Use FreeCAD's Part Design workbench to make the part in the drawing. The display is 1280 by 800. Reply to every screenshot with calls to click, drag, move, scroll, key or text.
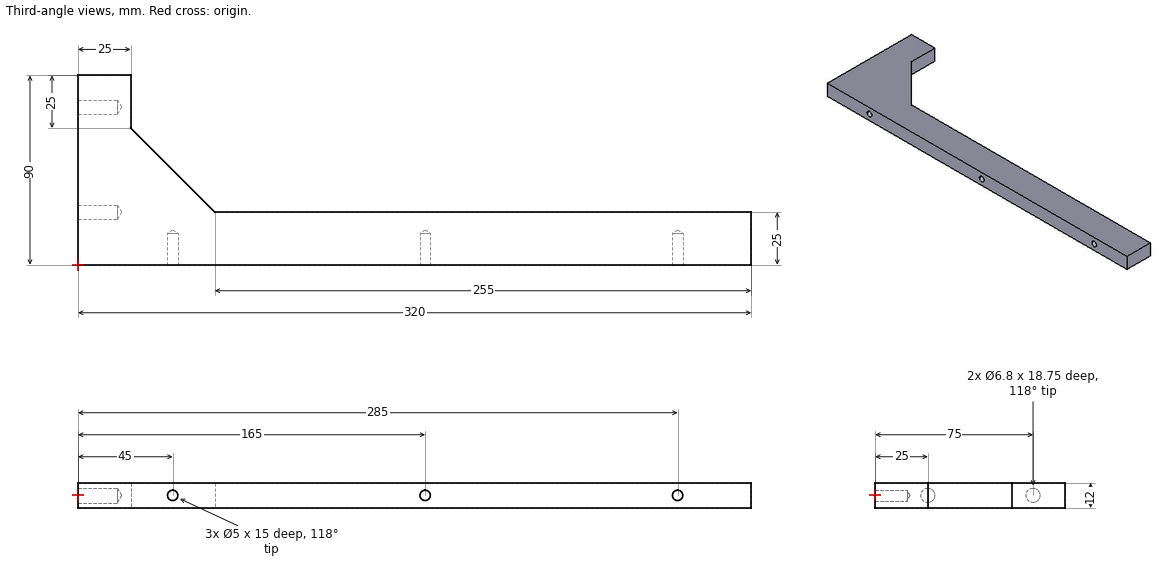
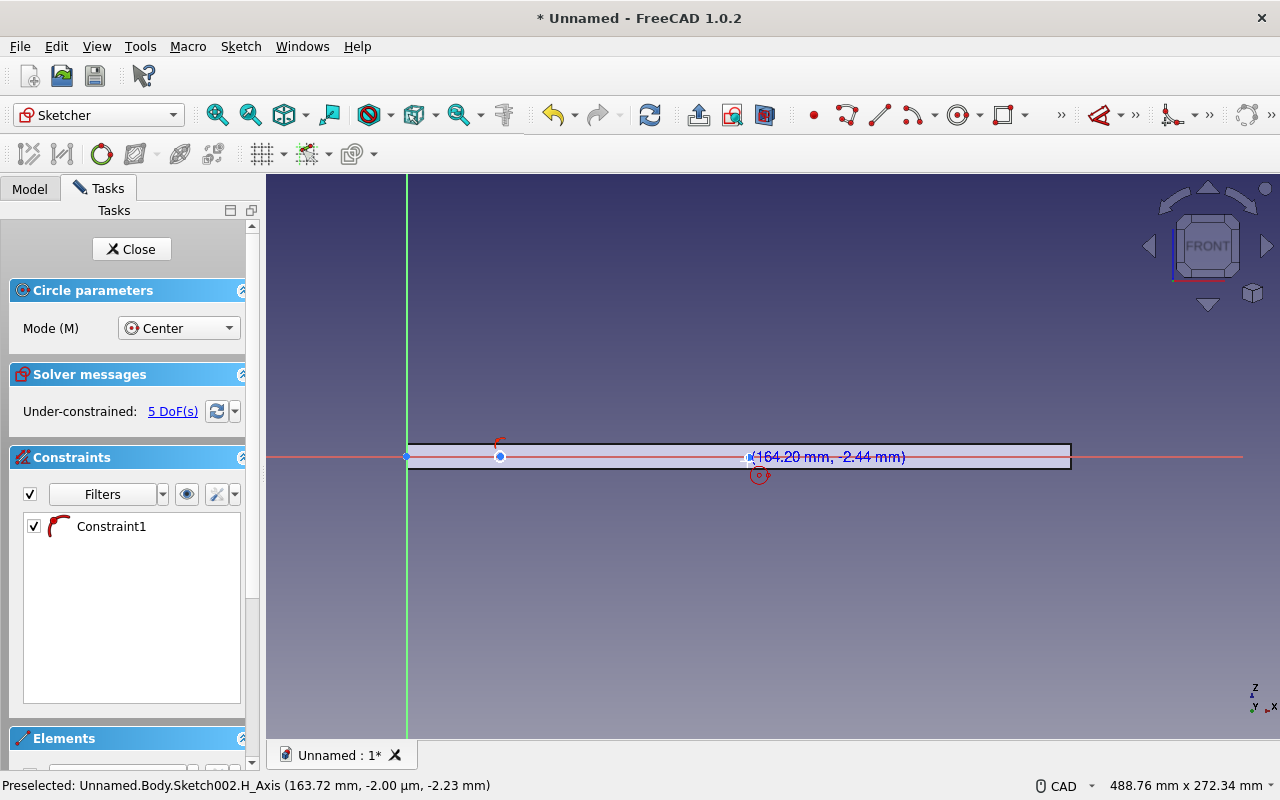
scroll(998, 457, up, 8)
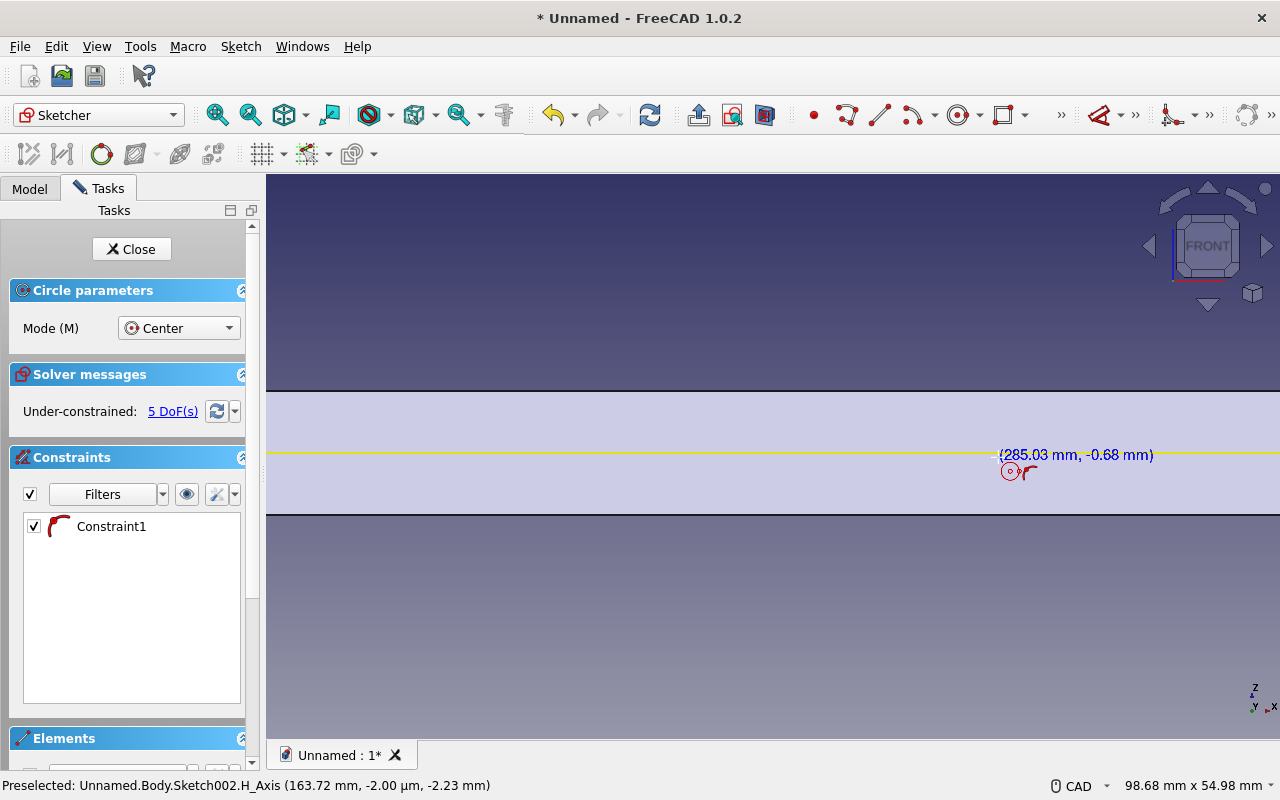
scroll(998, 457, down, 8)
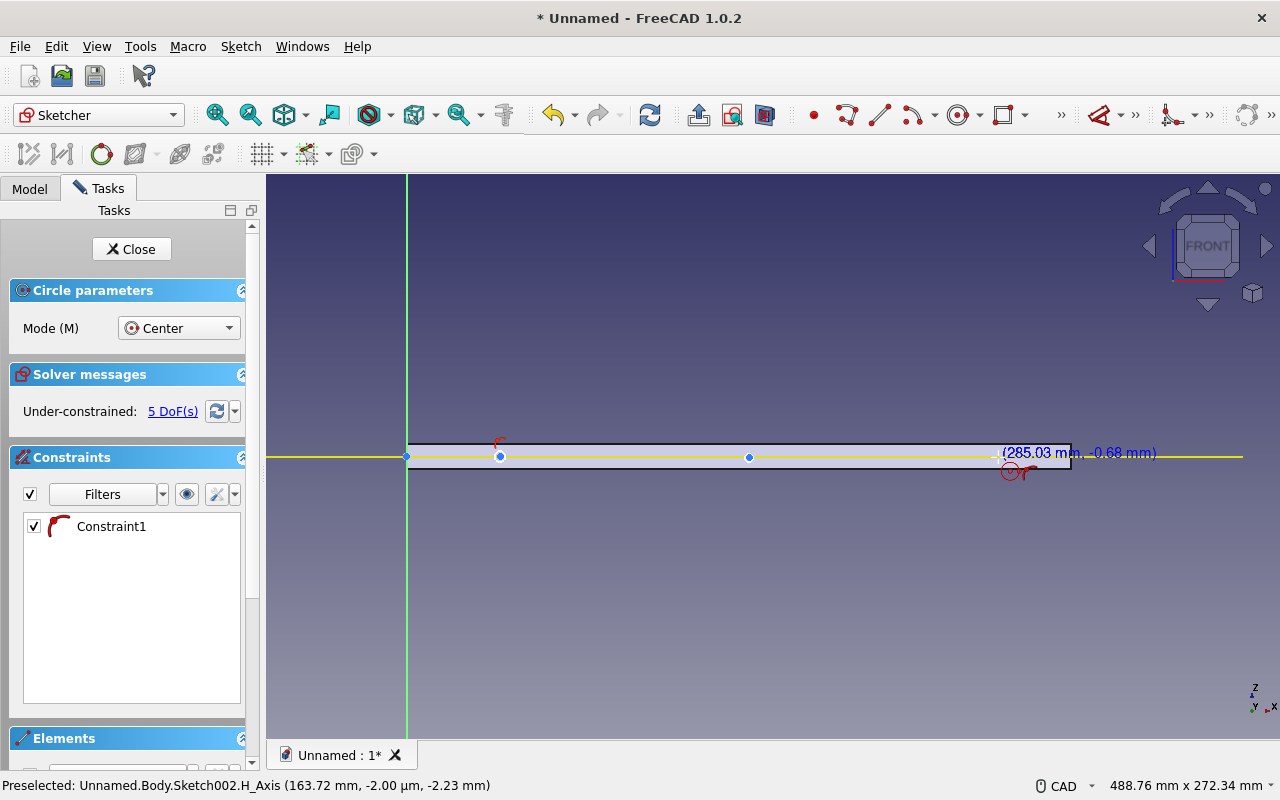
click(998, 457)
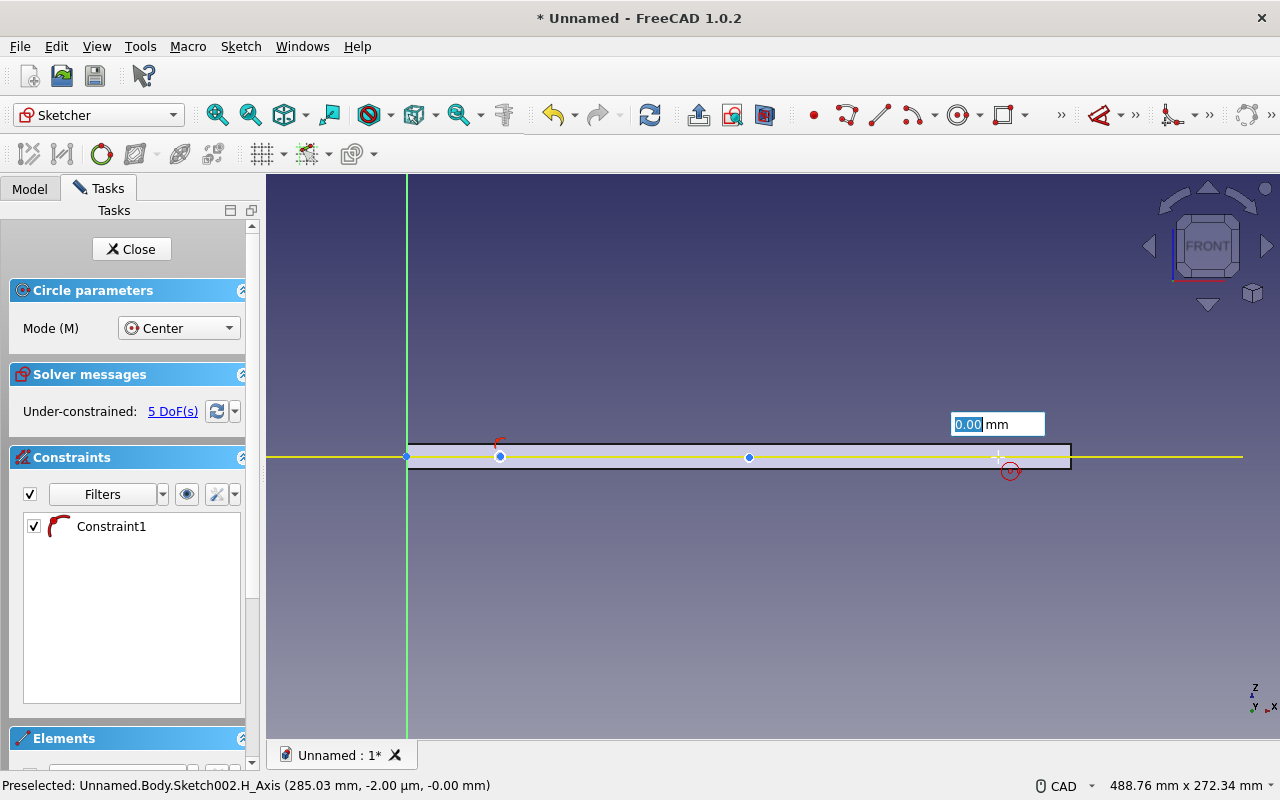
scroll(996, 461, up, 6)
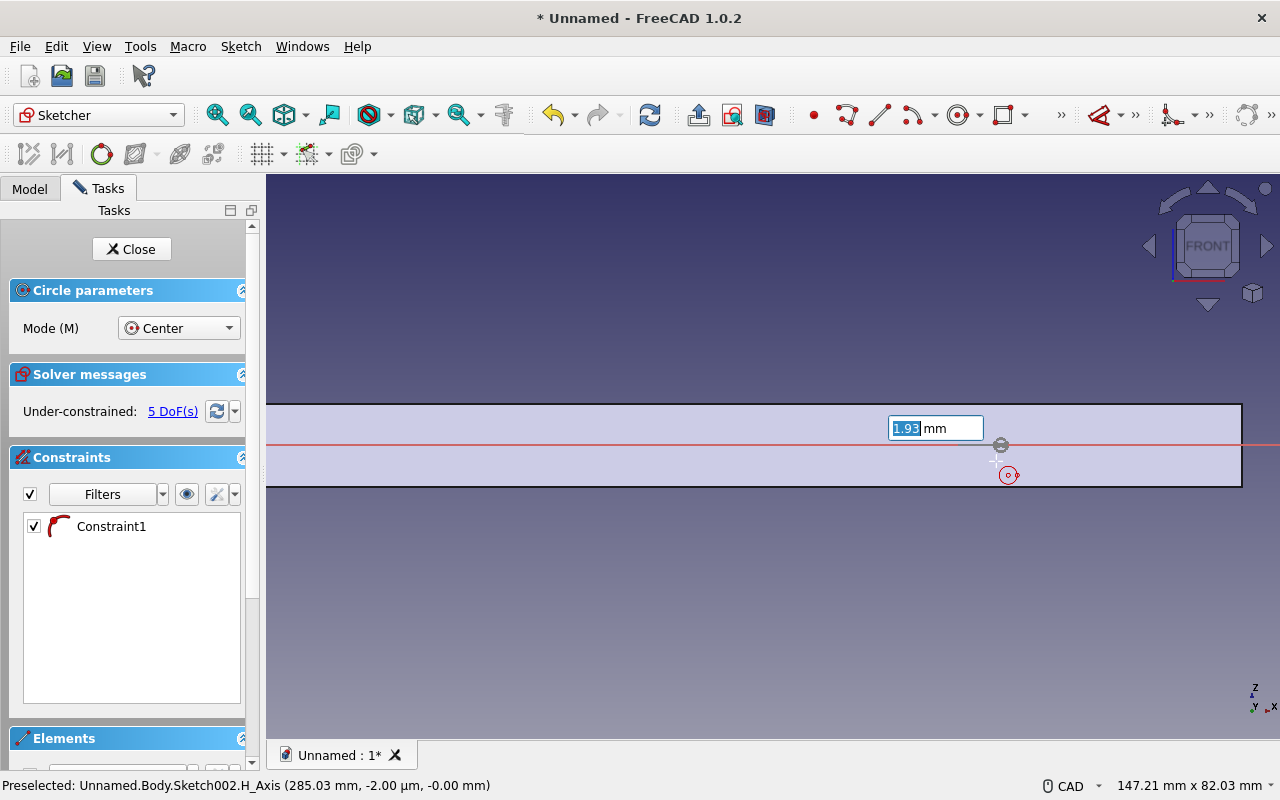
click(995, 461)
key(Escape)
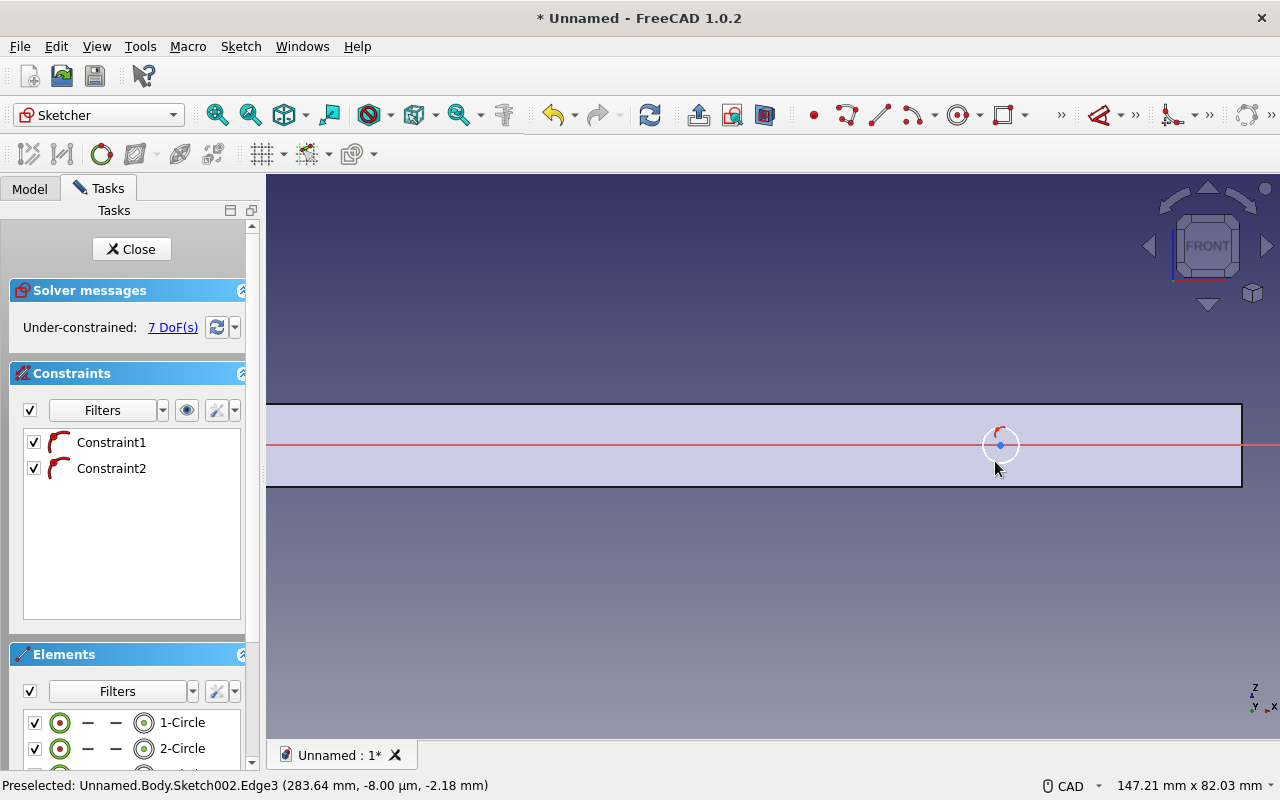
scroll(996, 461, down, 6)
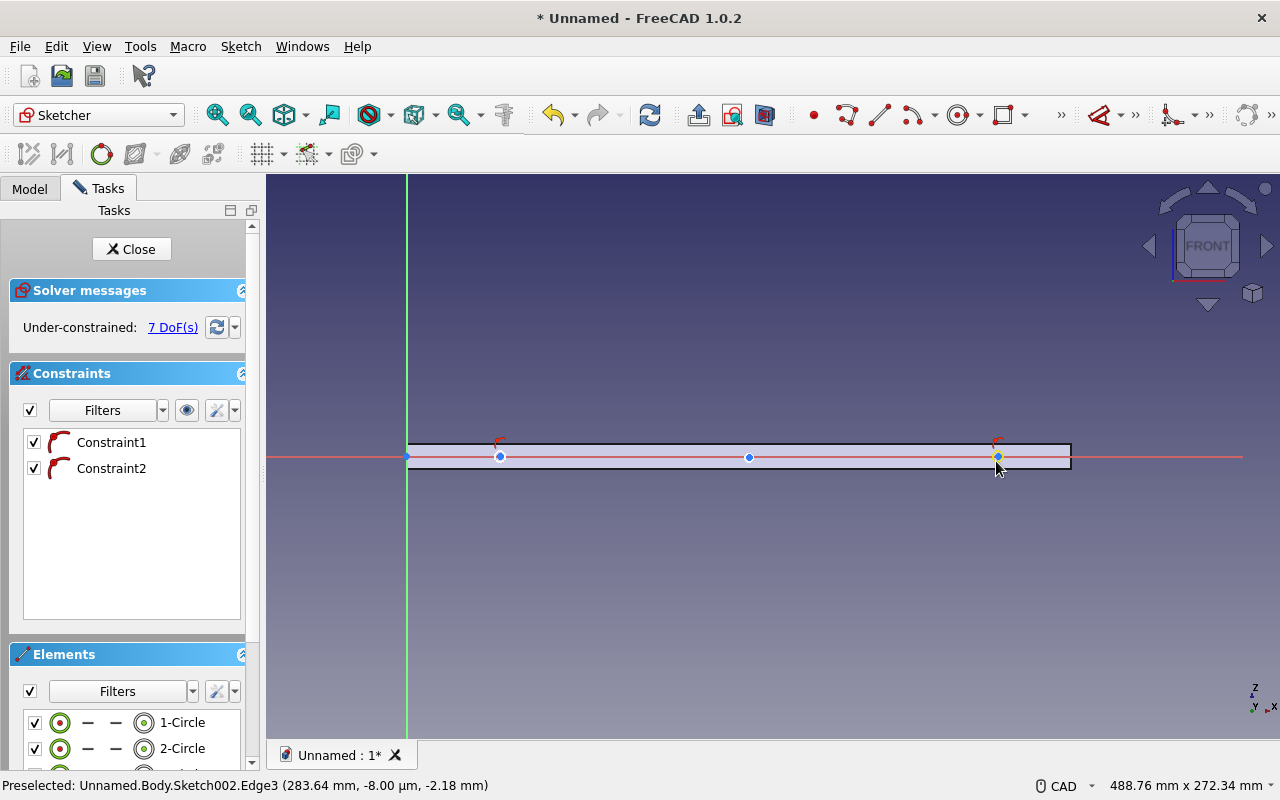
scroll(504, 453, up, 7)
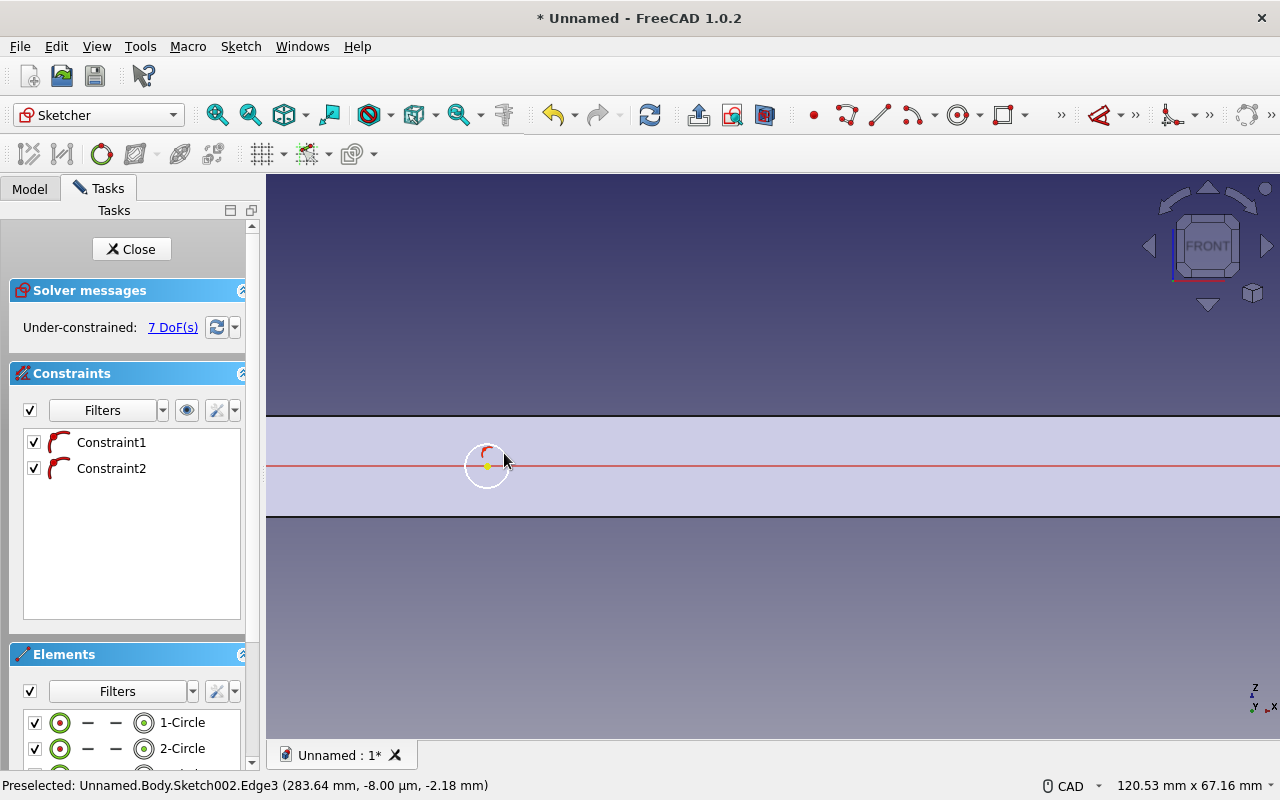
click(502, 451)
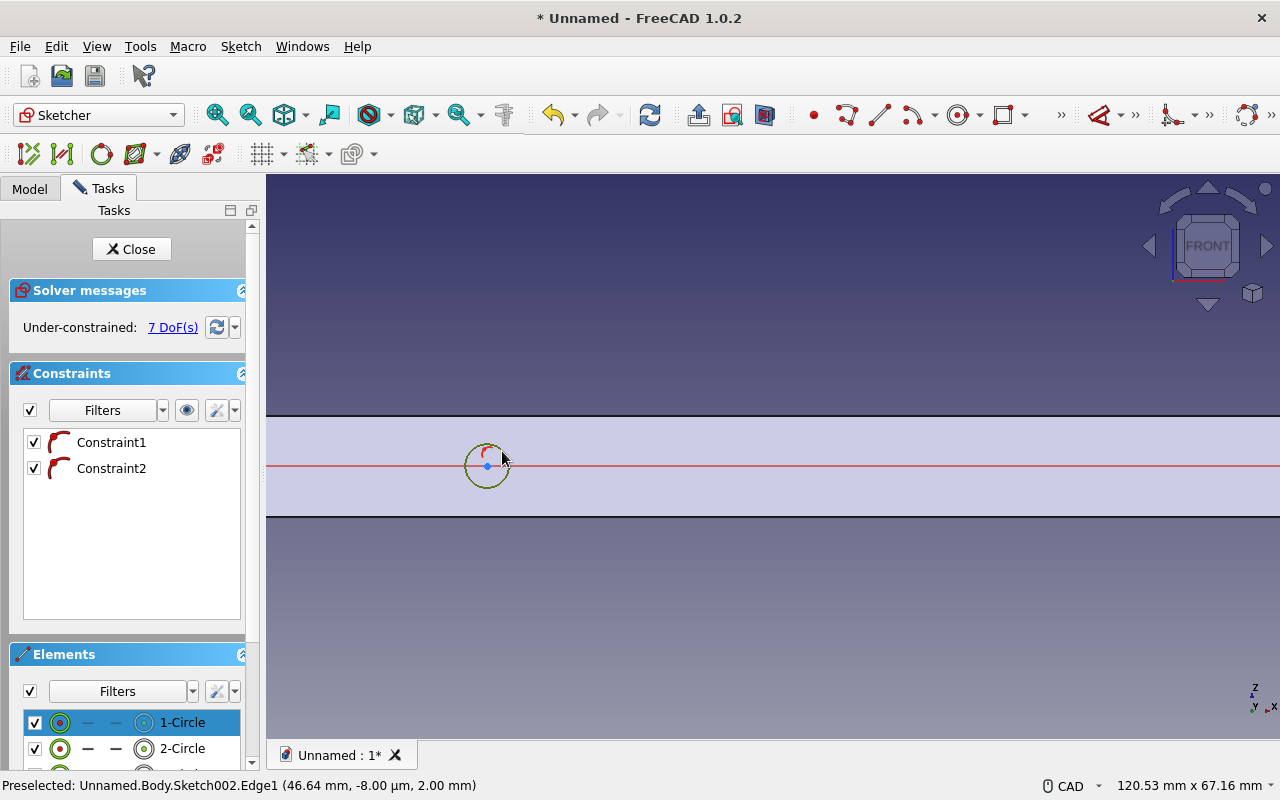
scroll(504, 453, down, 7)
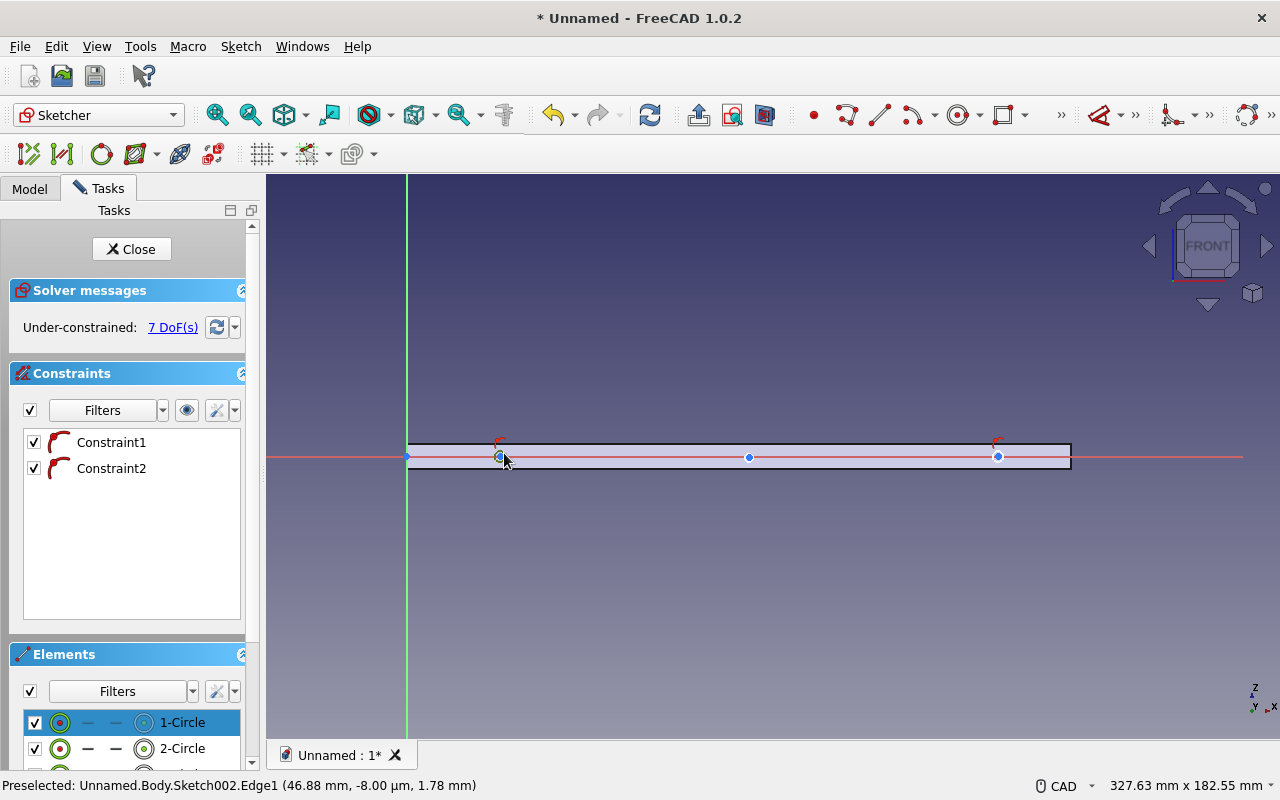
scroll(746, 461, up, 7)